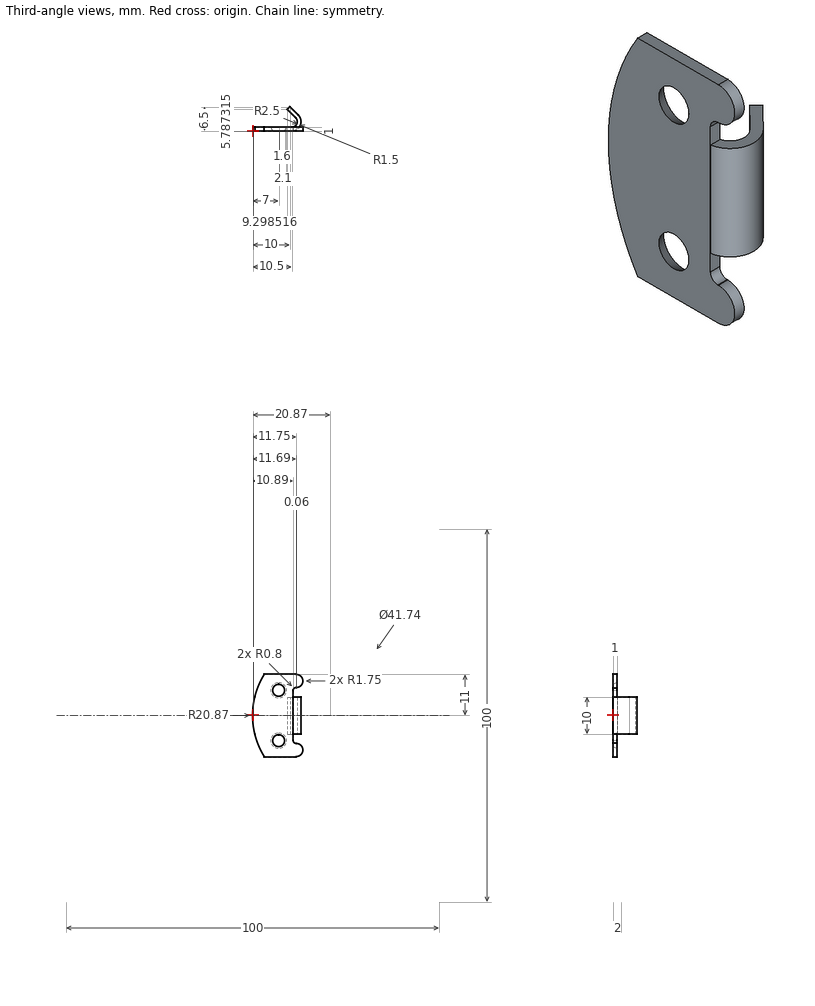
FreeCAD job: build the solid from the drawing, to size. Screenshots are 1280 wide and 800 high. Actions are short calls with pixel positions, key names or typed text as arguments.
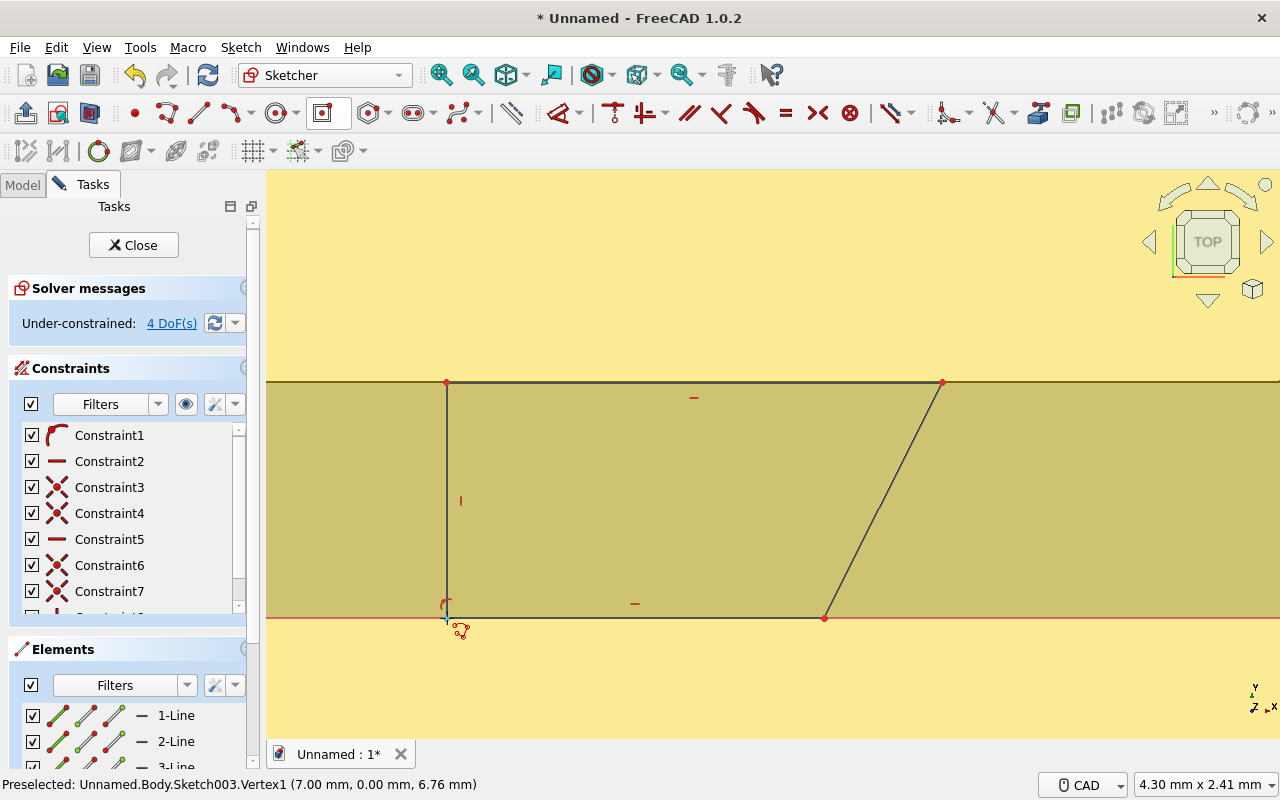
click(200, 114)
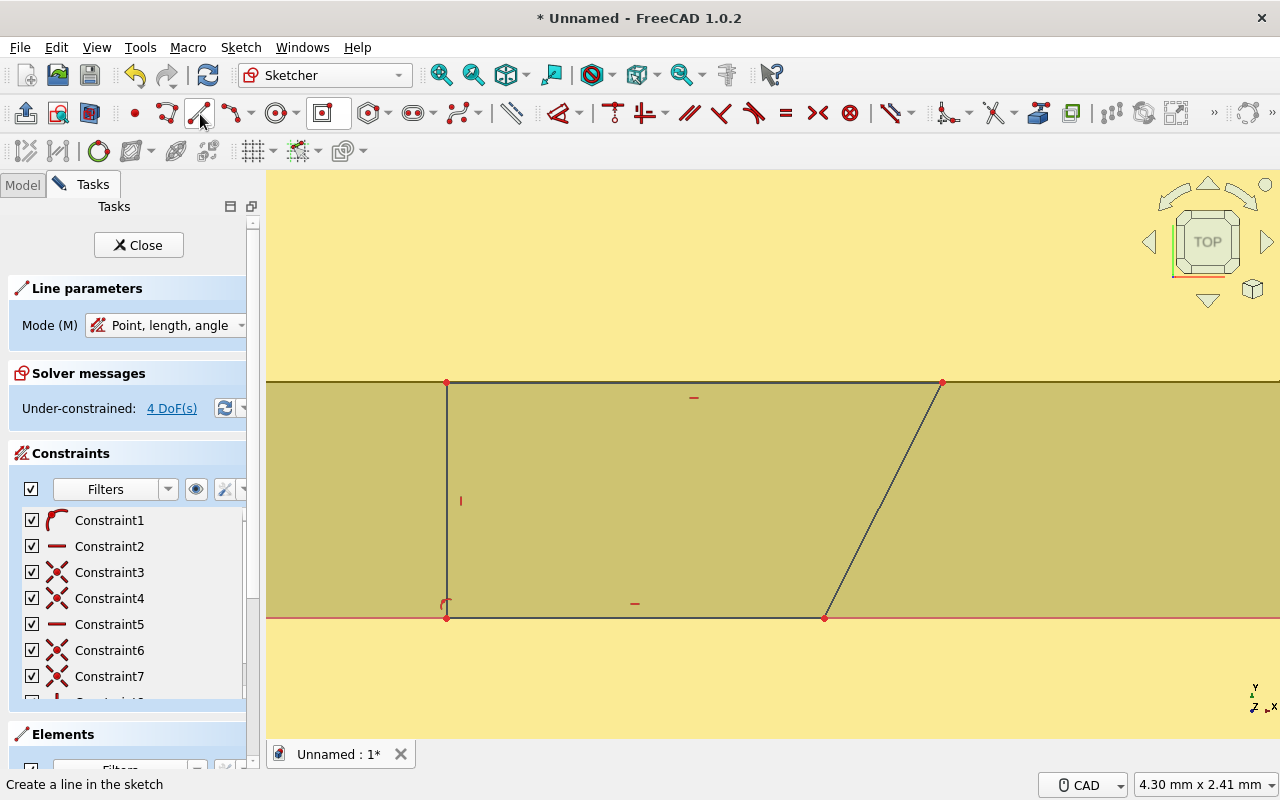
click(447, 359)
click(447, 288)
key(Escape)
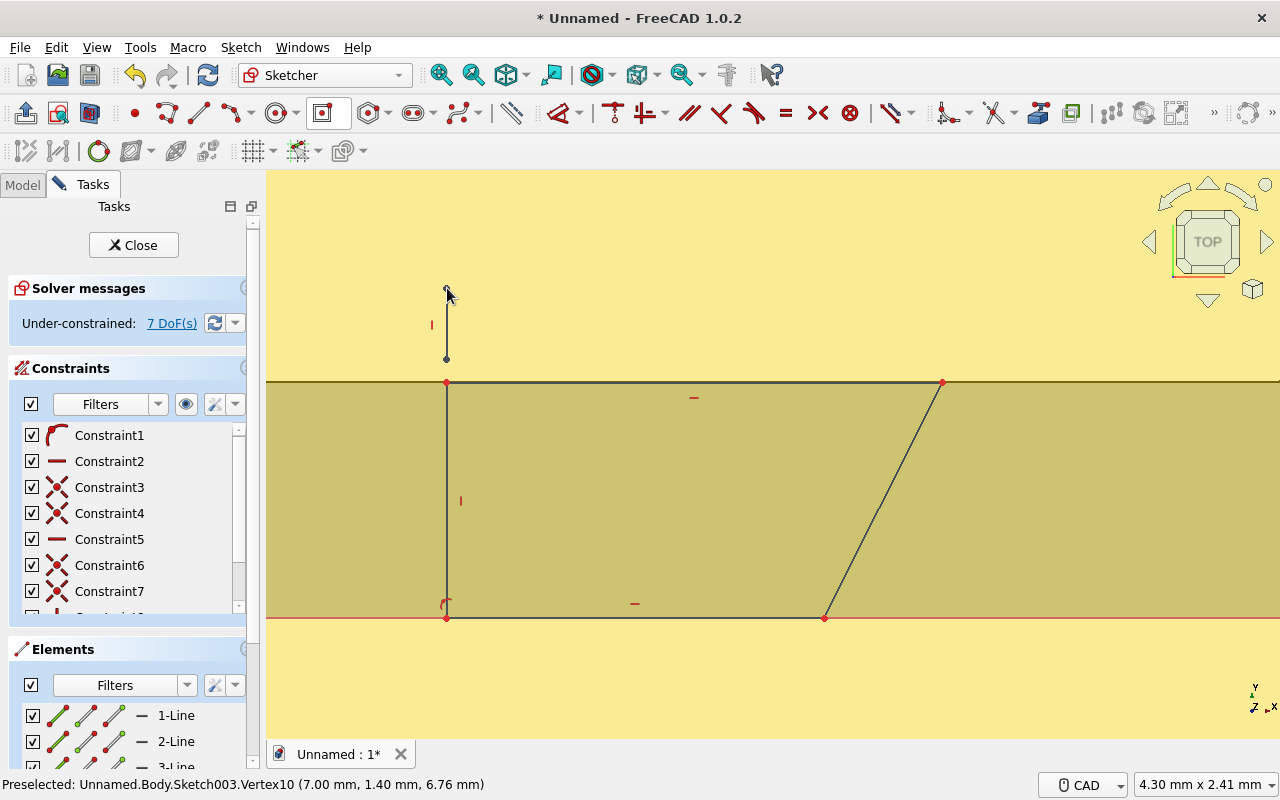
click(447, 339)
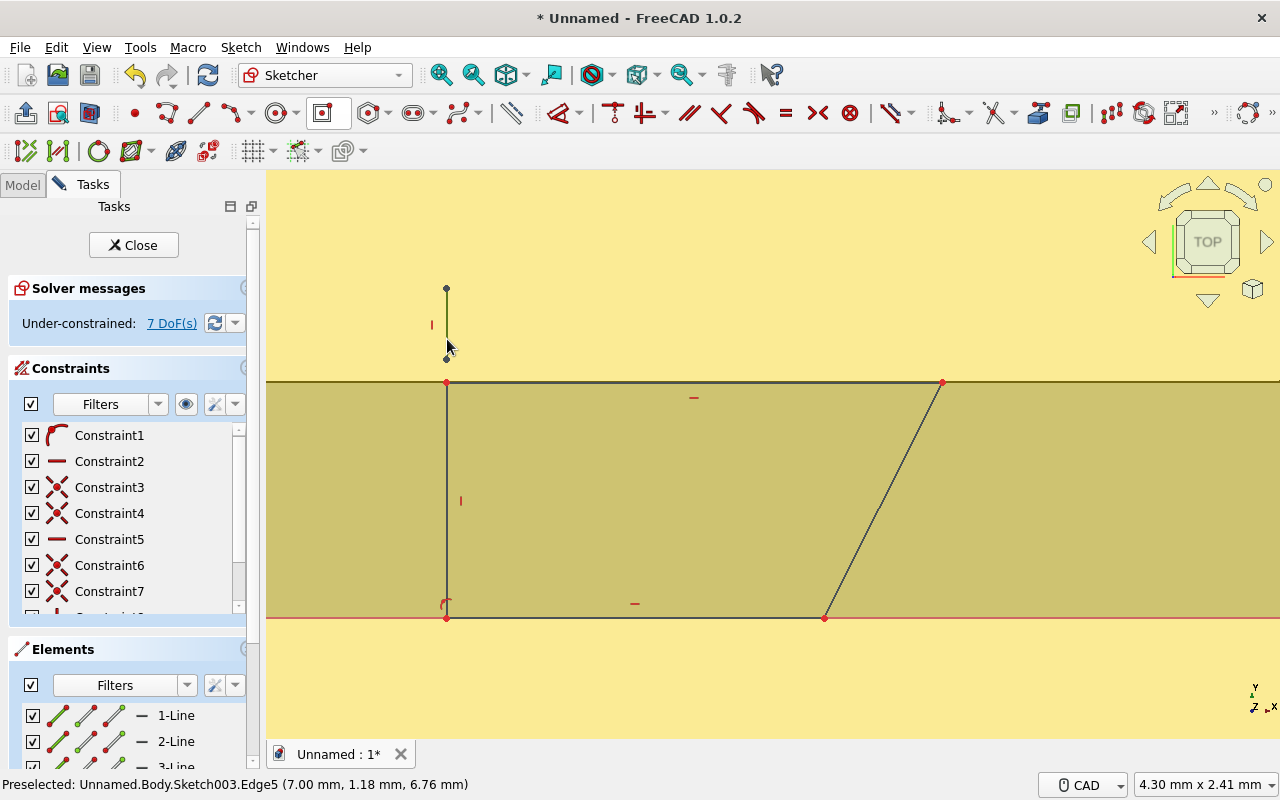
click(512, 114)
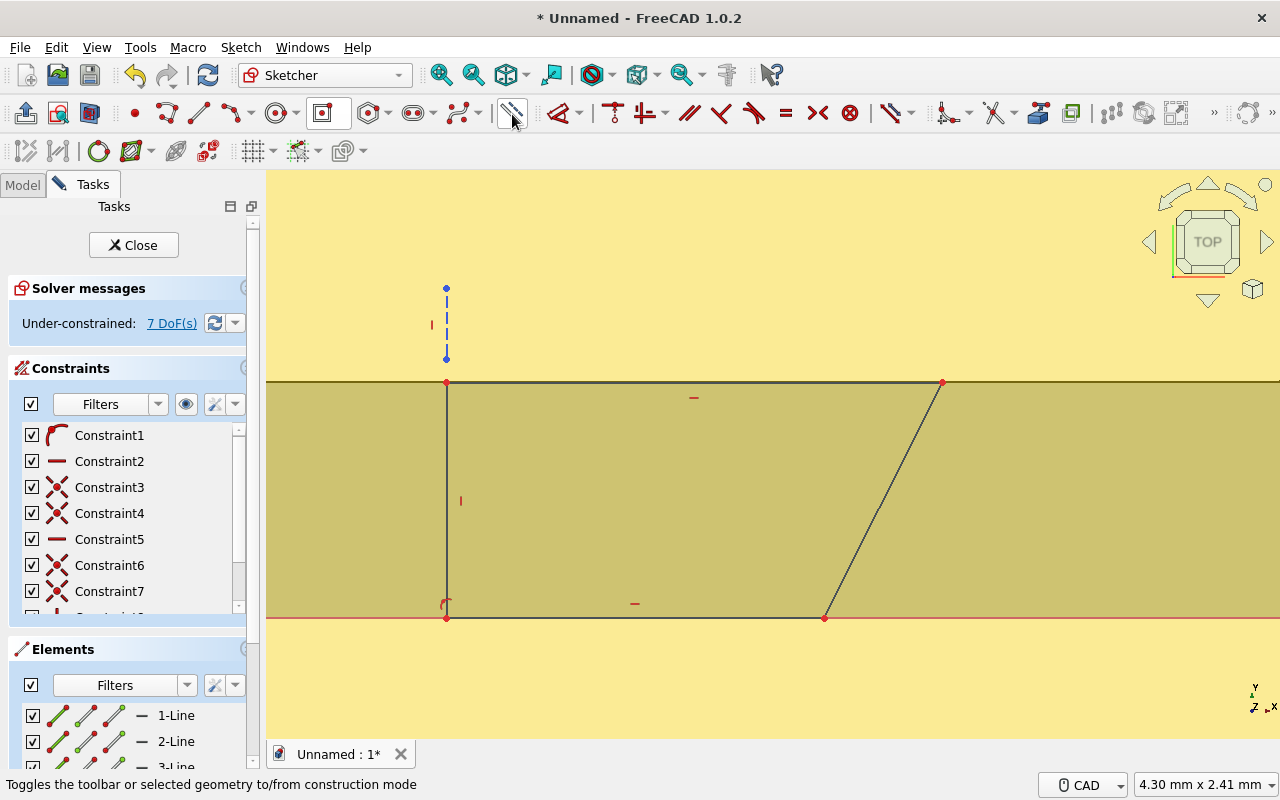
click(558, 114)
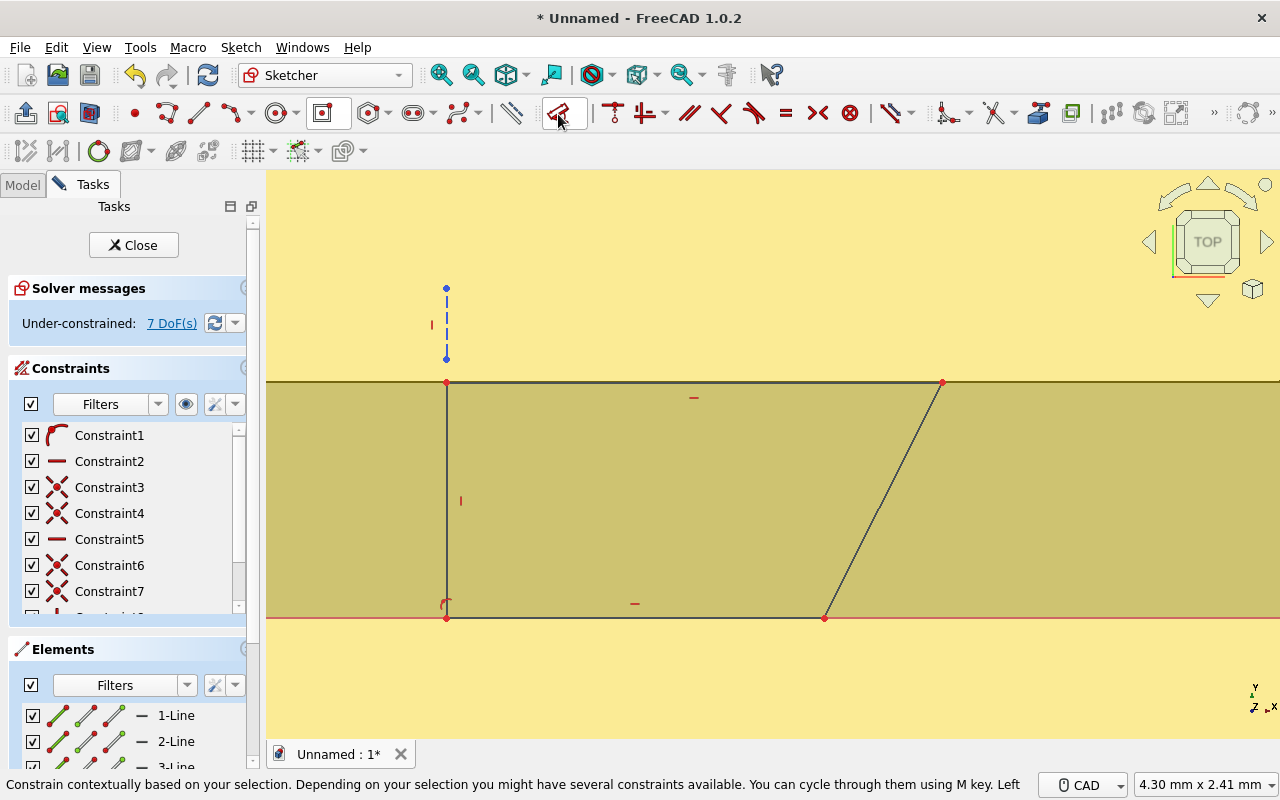
click(447, 454)
click(413, 501)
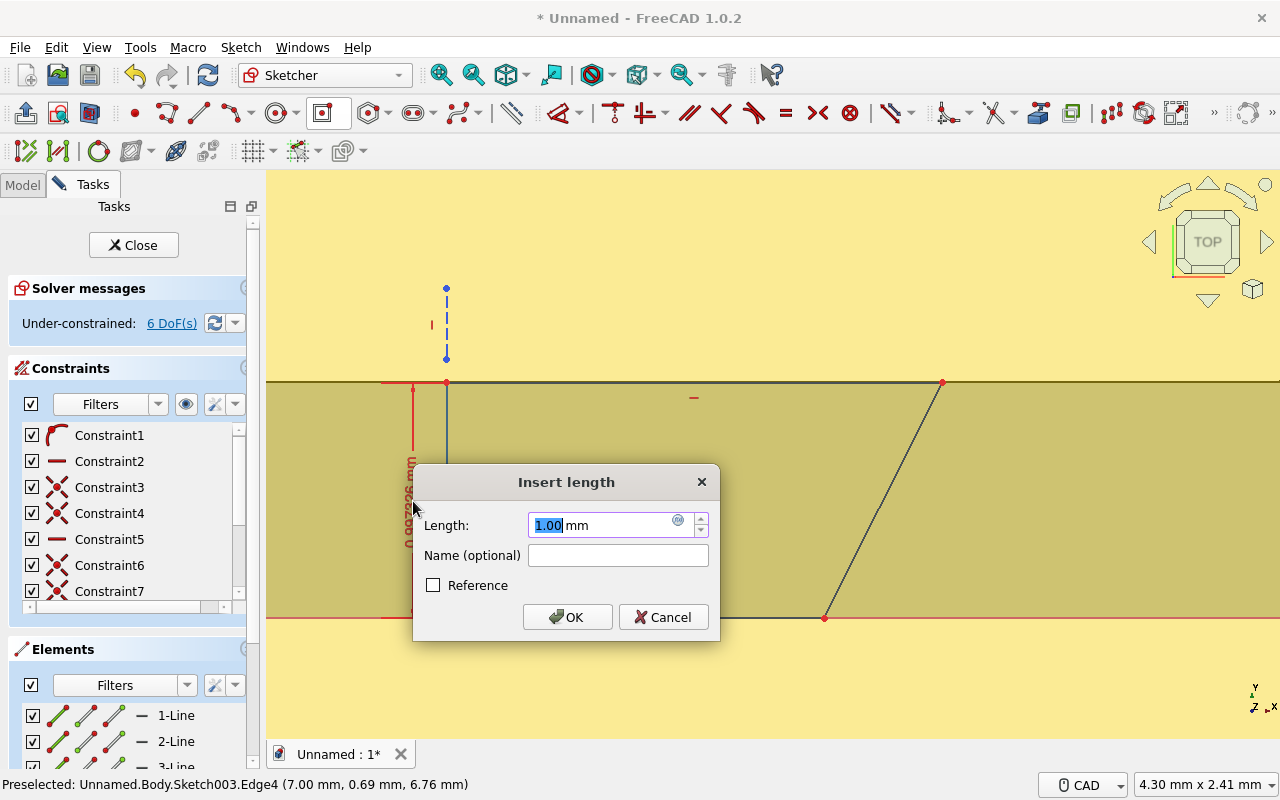
text(1)
key(Return)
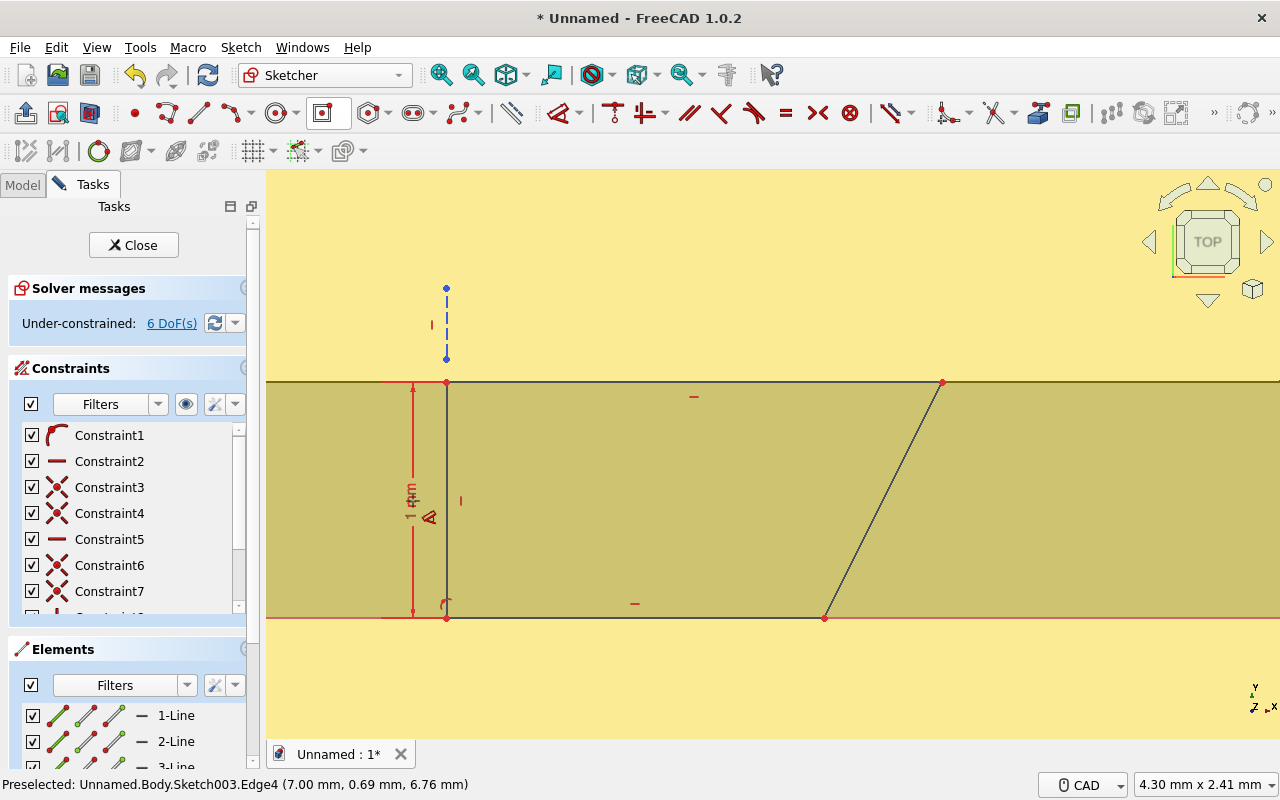
click(447, 618)
click(370, 652)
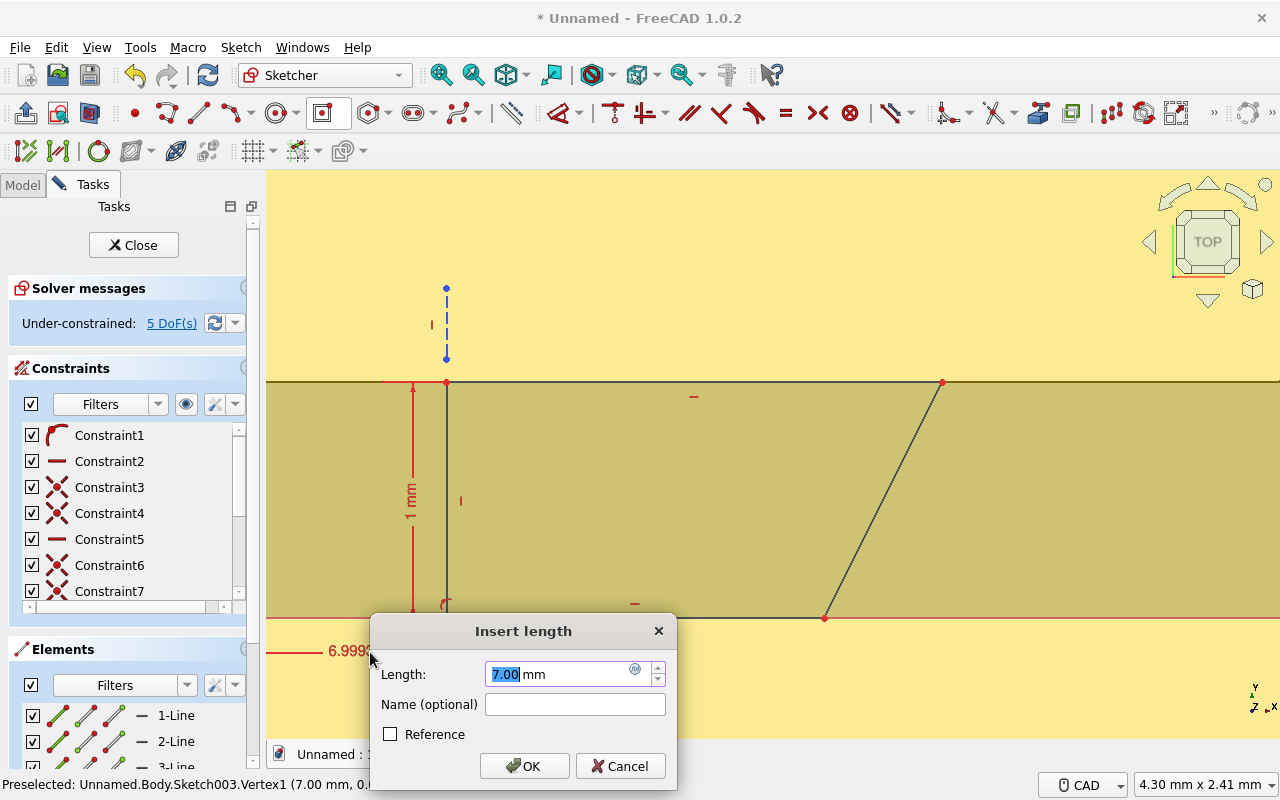
text(7)
key(Return)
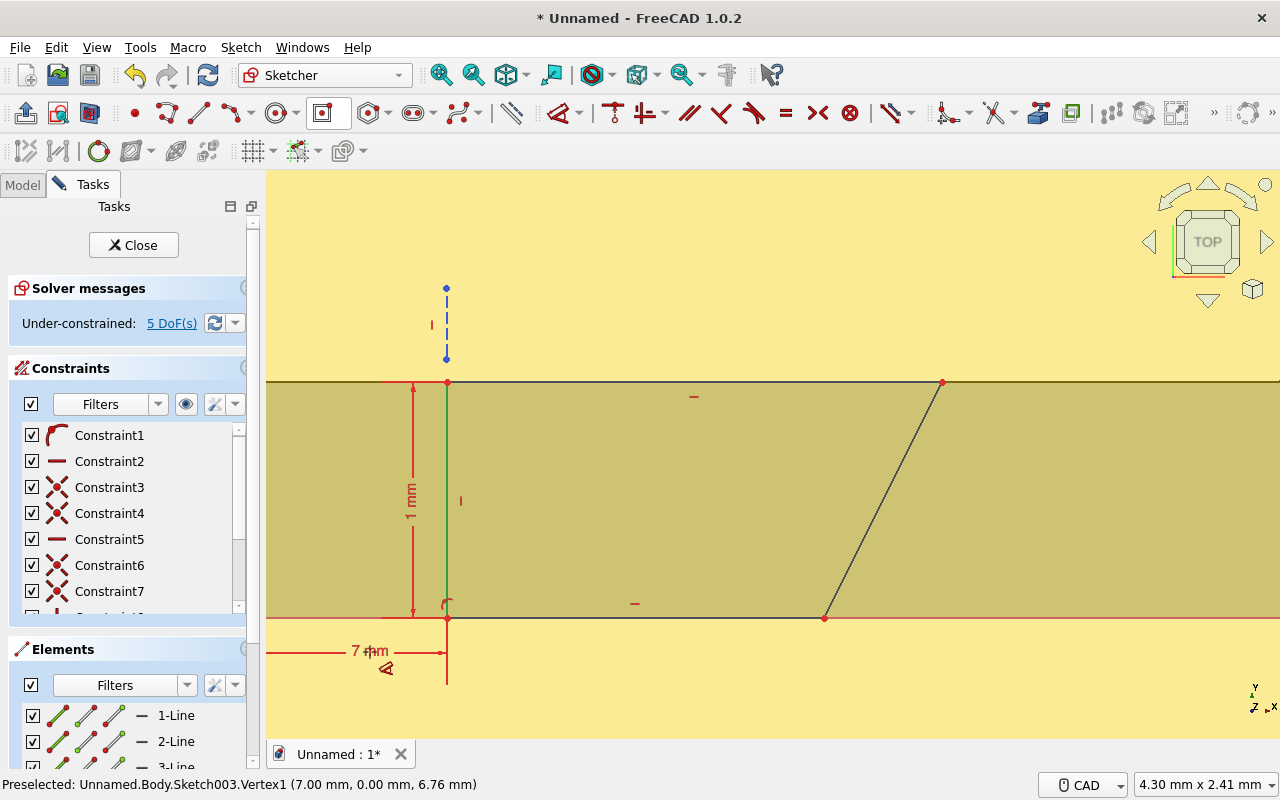
click(447, 360)
click(370, 326)